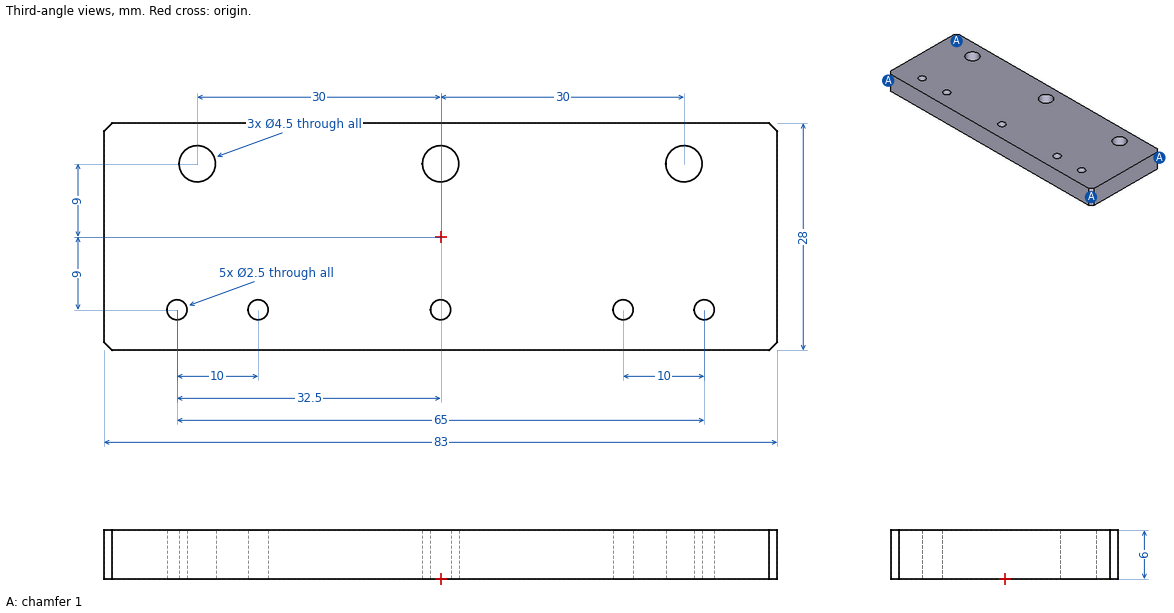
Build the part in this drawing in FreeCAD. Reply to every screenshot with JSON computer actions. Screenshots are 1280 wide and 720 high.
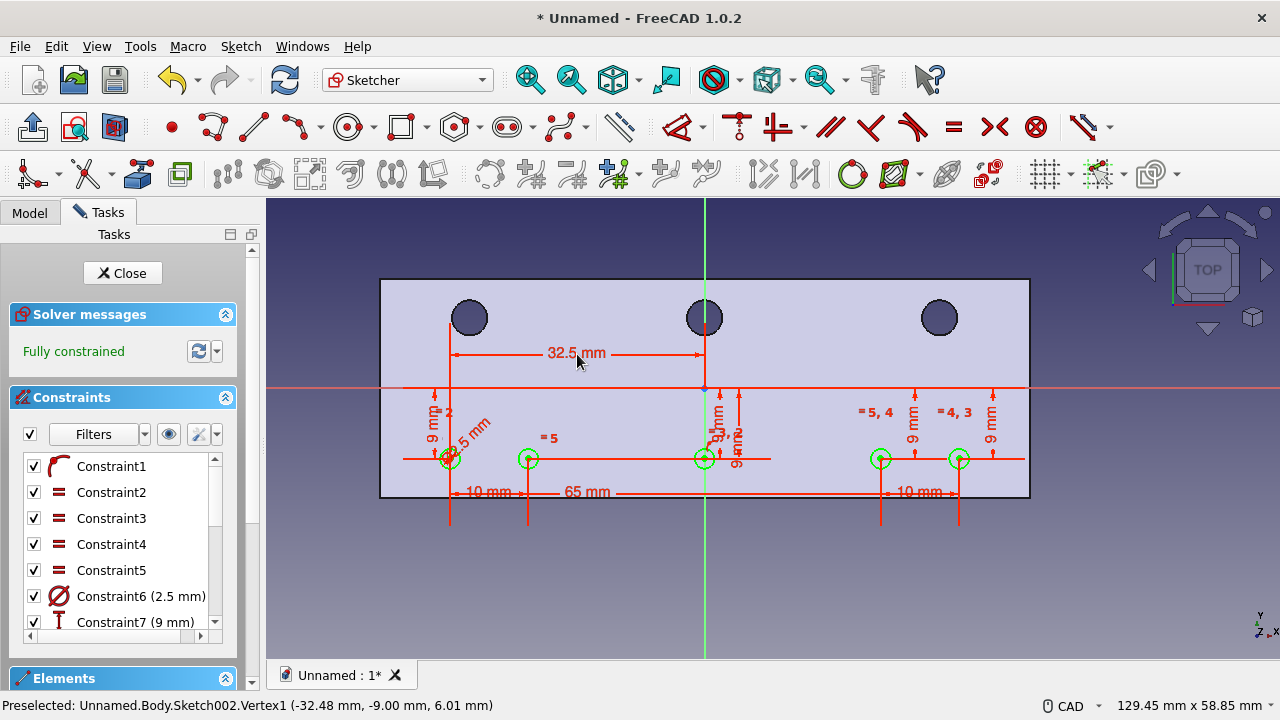
{"action": "left_click", "coordinate": [123, 273]}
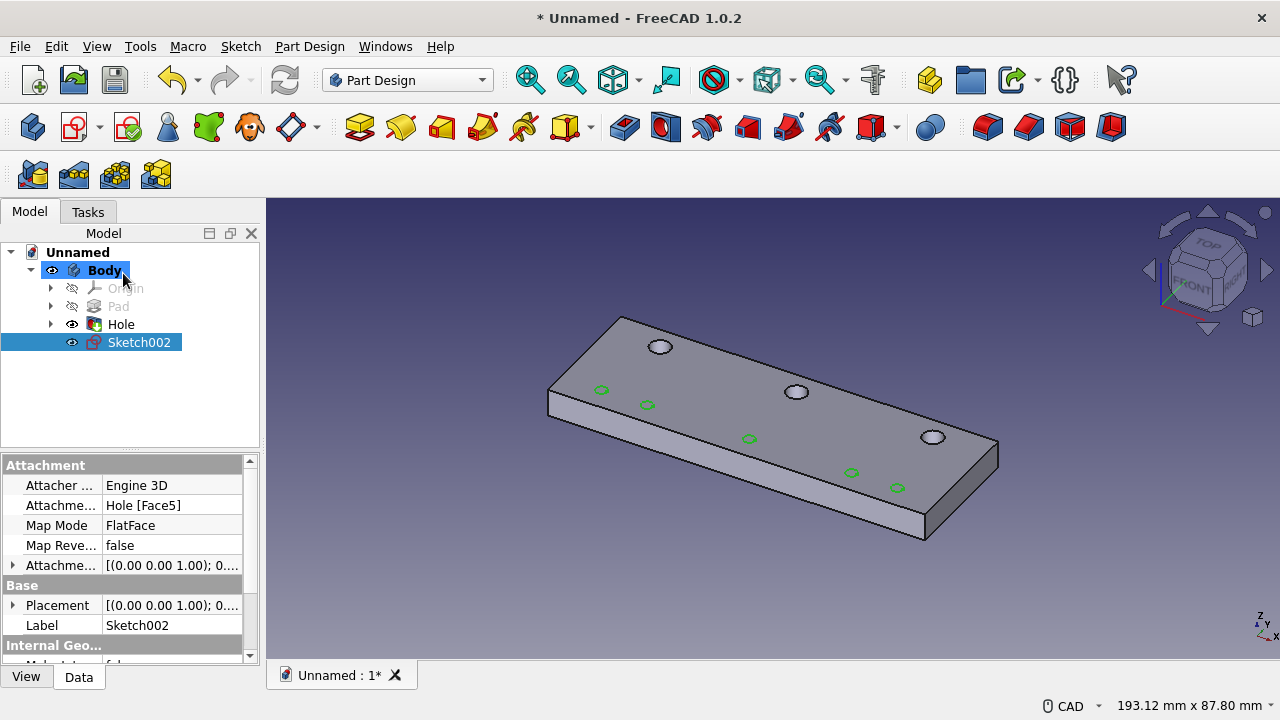
{"action": "left_click", "coordinate": [666, 128]}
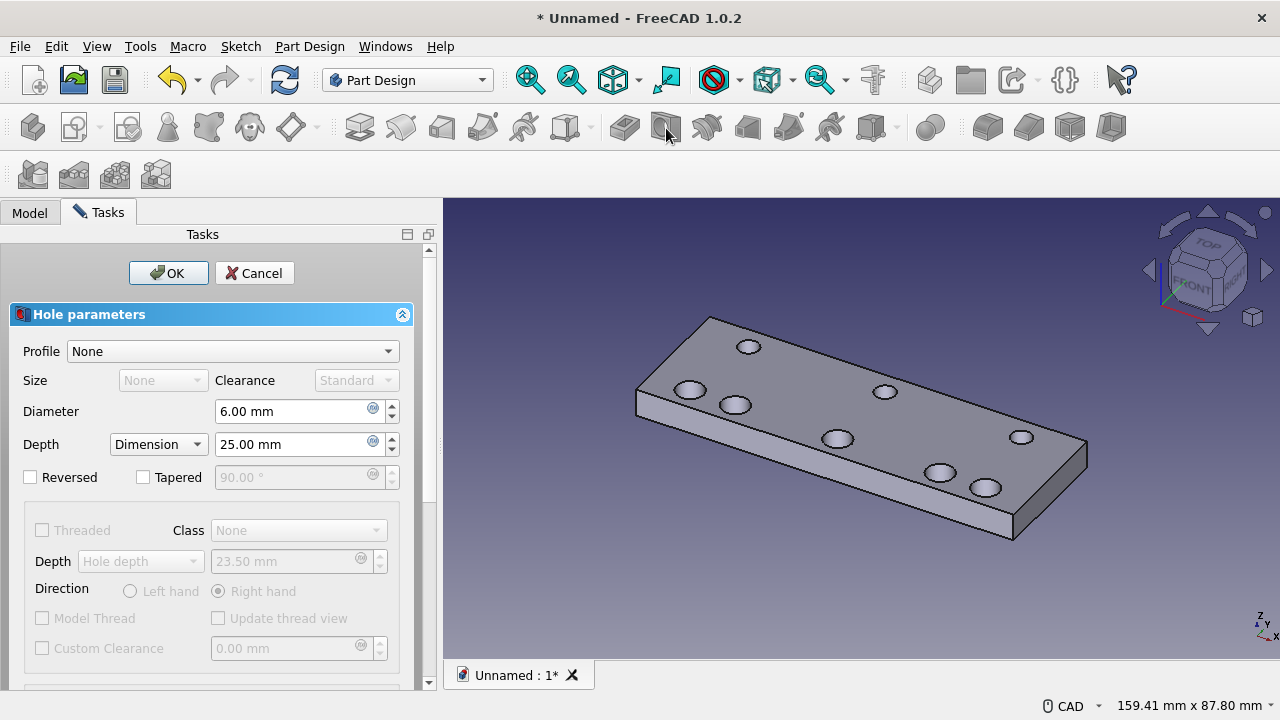
{"action": "triple_click", "coordinate": [300, 412]}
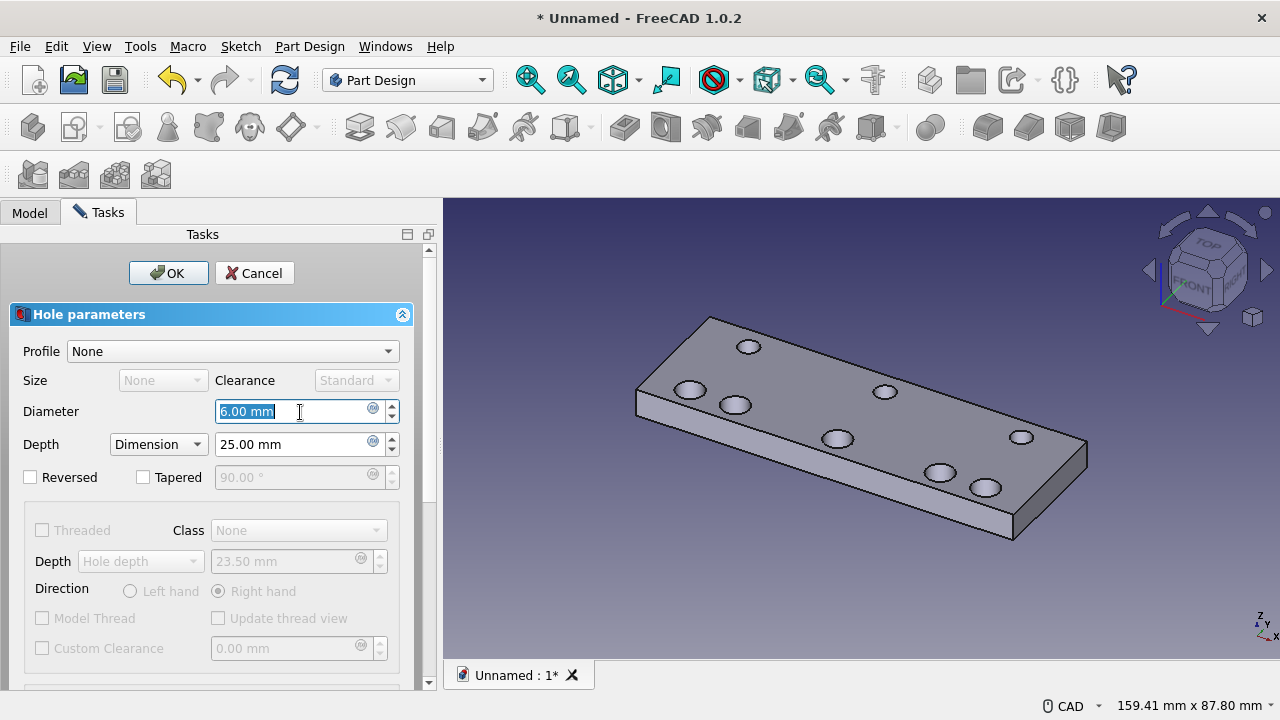
{"action": "type", "text": "2.5"}
{"action": "key", "text": "Tab"}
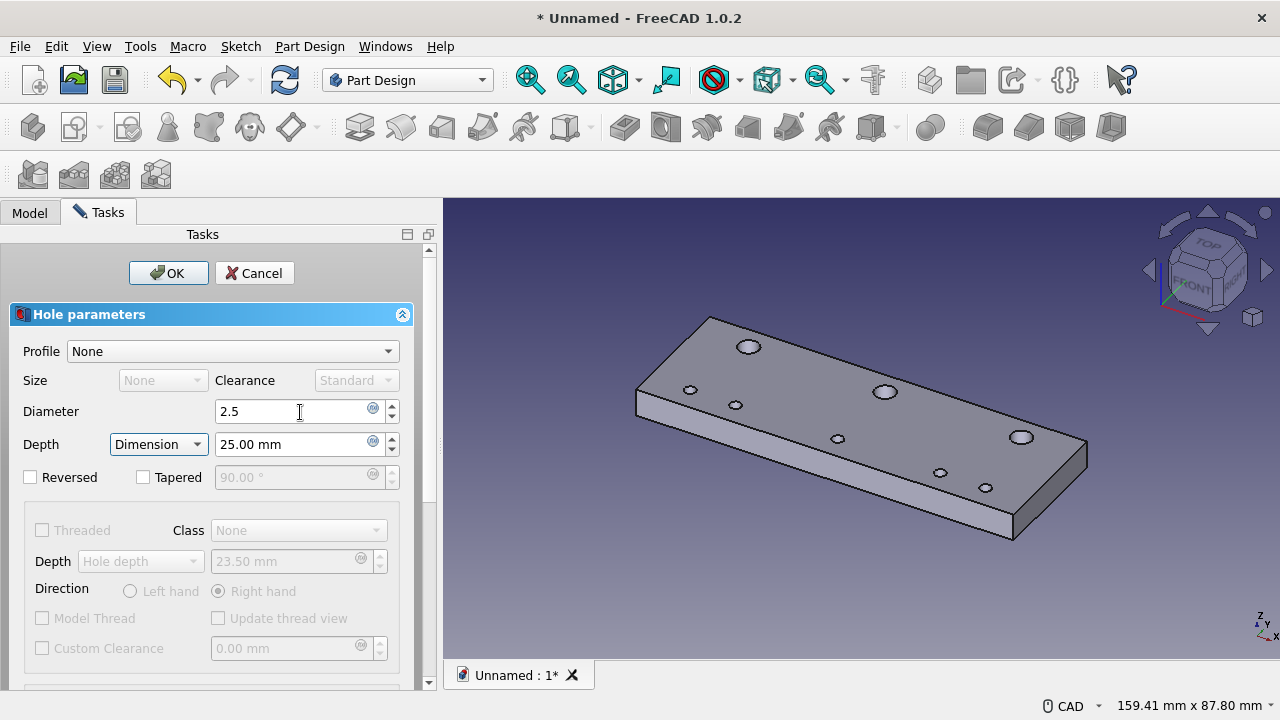
{"action": "left_click", "coordinate": [160, 444]}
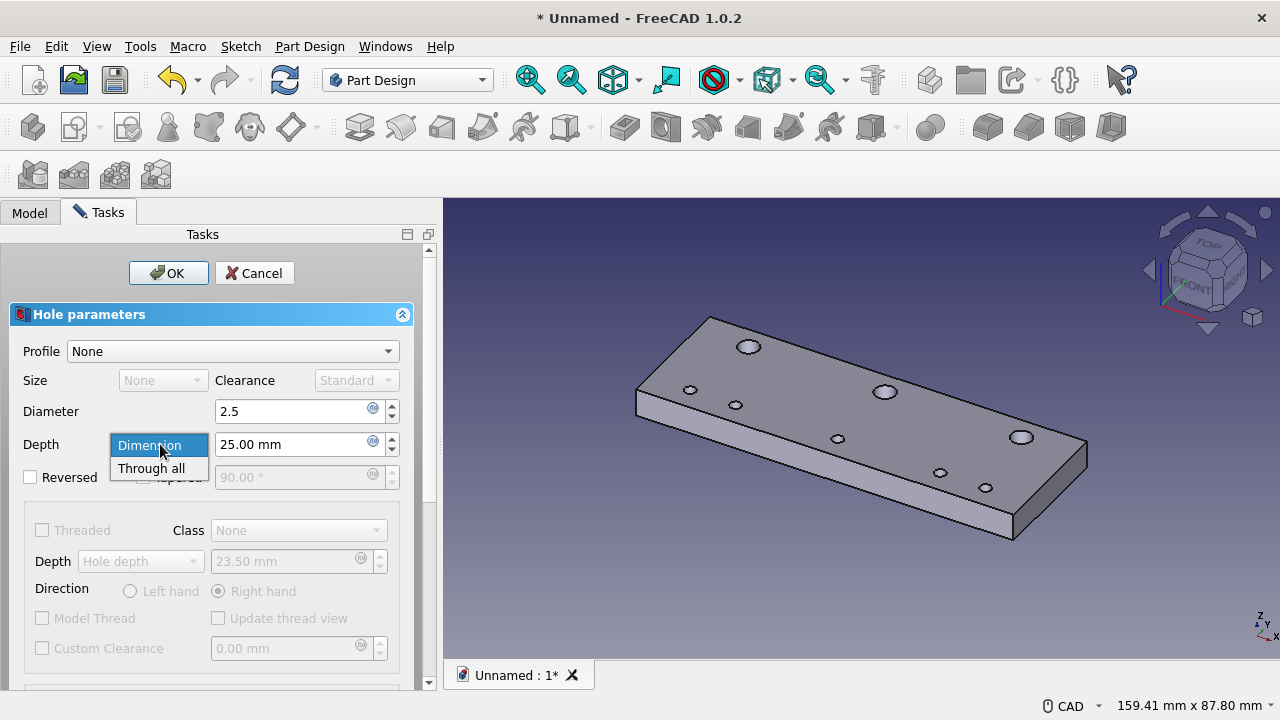
{"action": "left_click", "coordinate": [158, 468]}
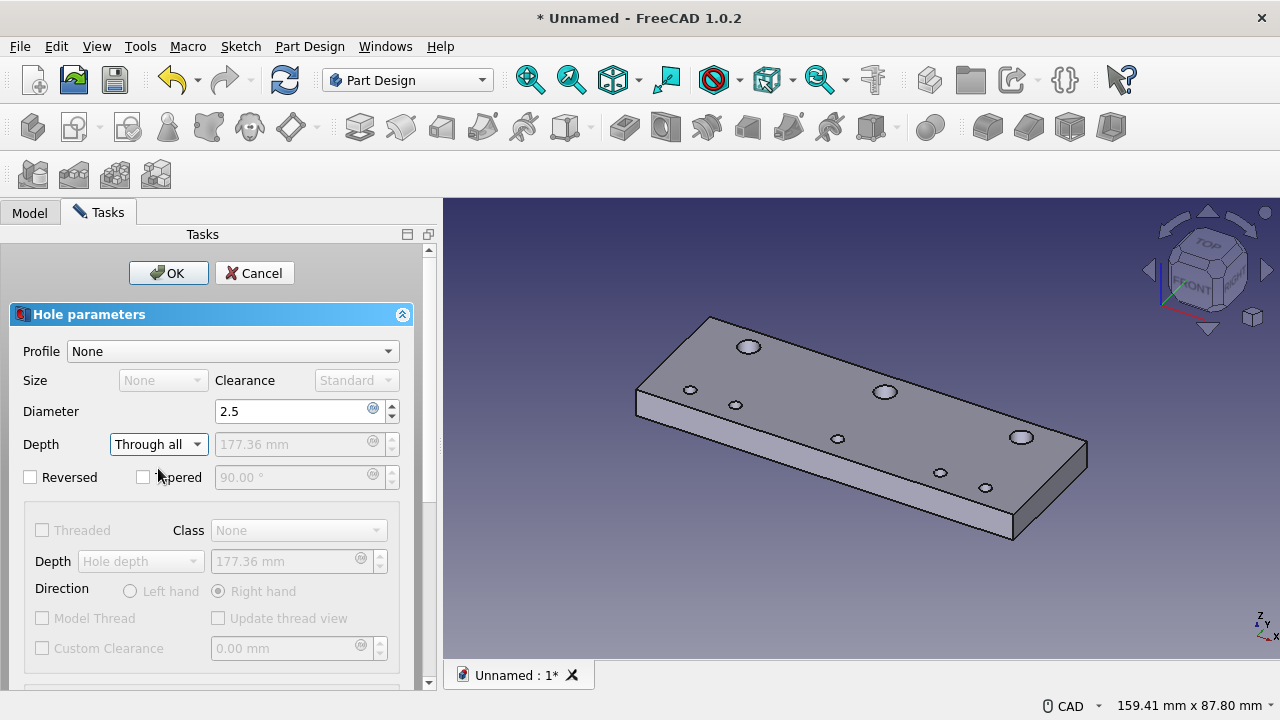
{"action": "left_click", "coordinate": [169, 273]}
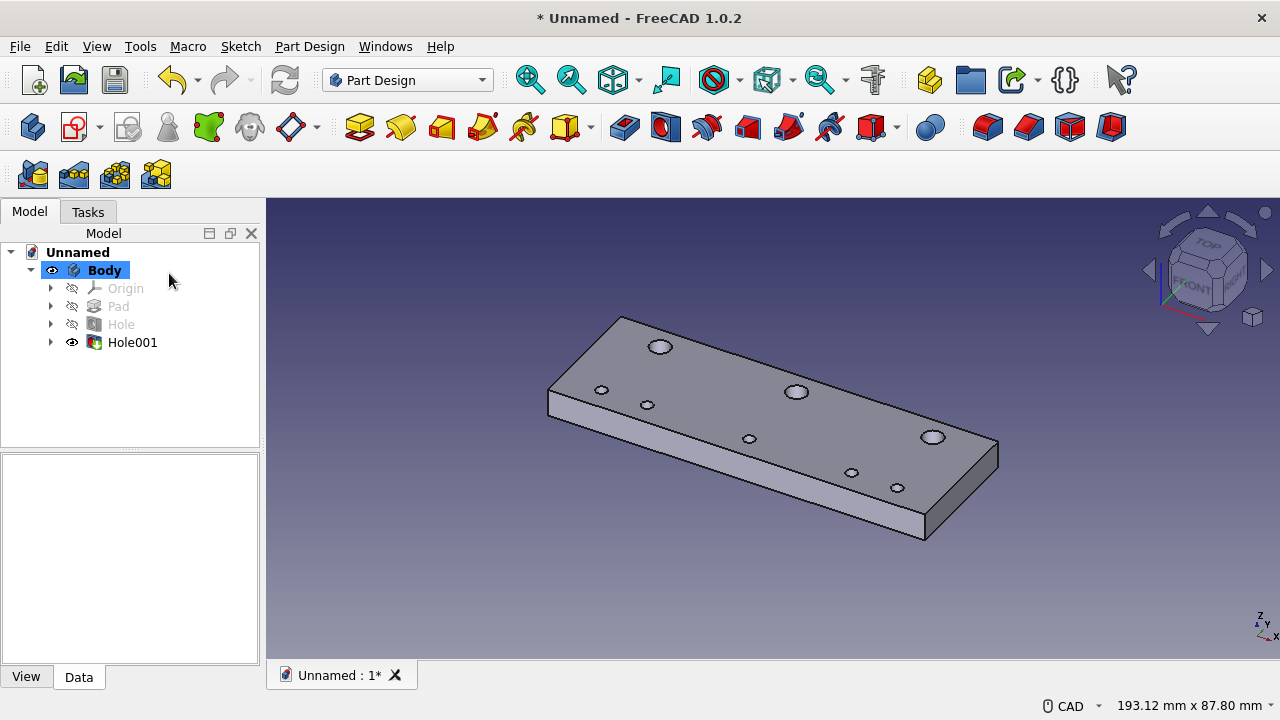
{"action": "left_click", "coordinate": [925, 527]}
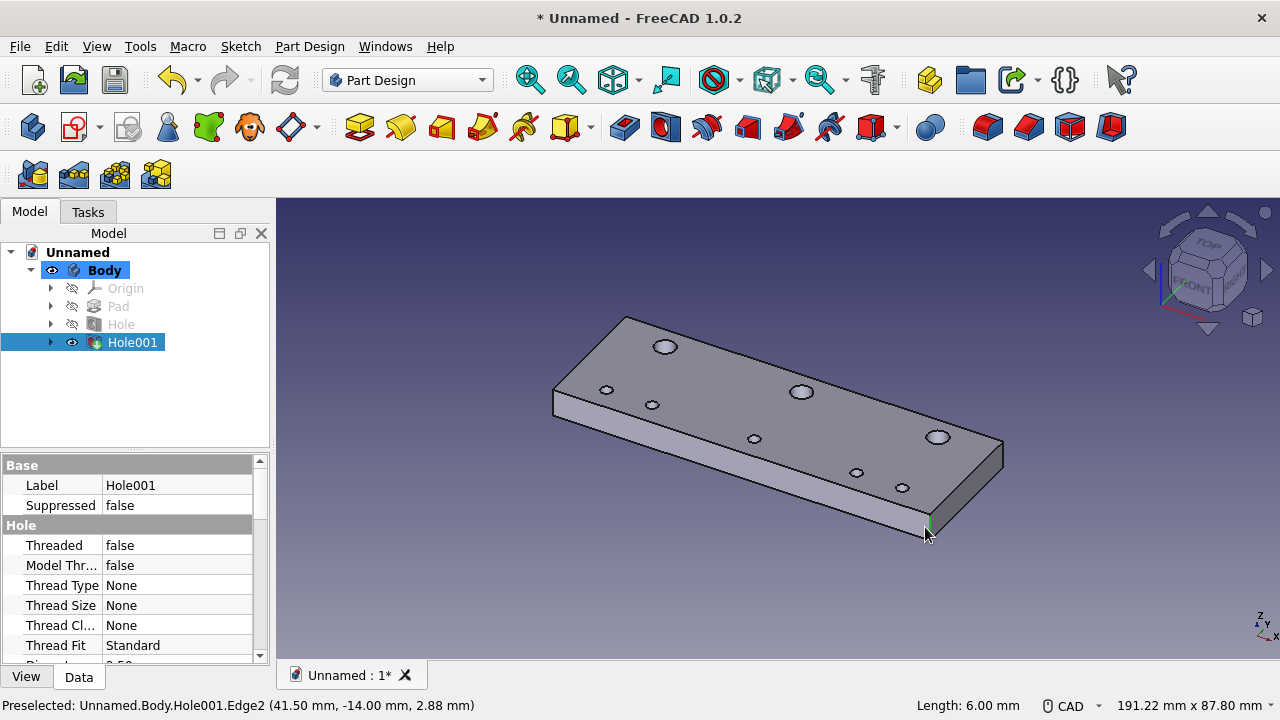
{"action": "key", "text": "0"}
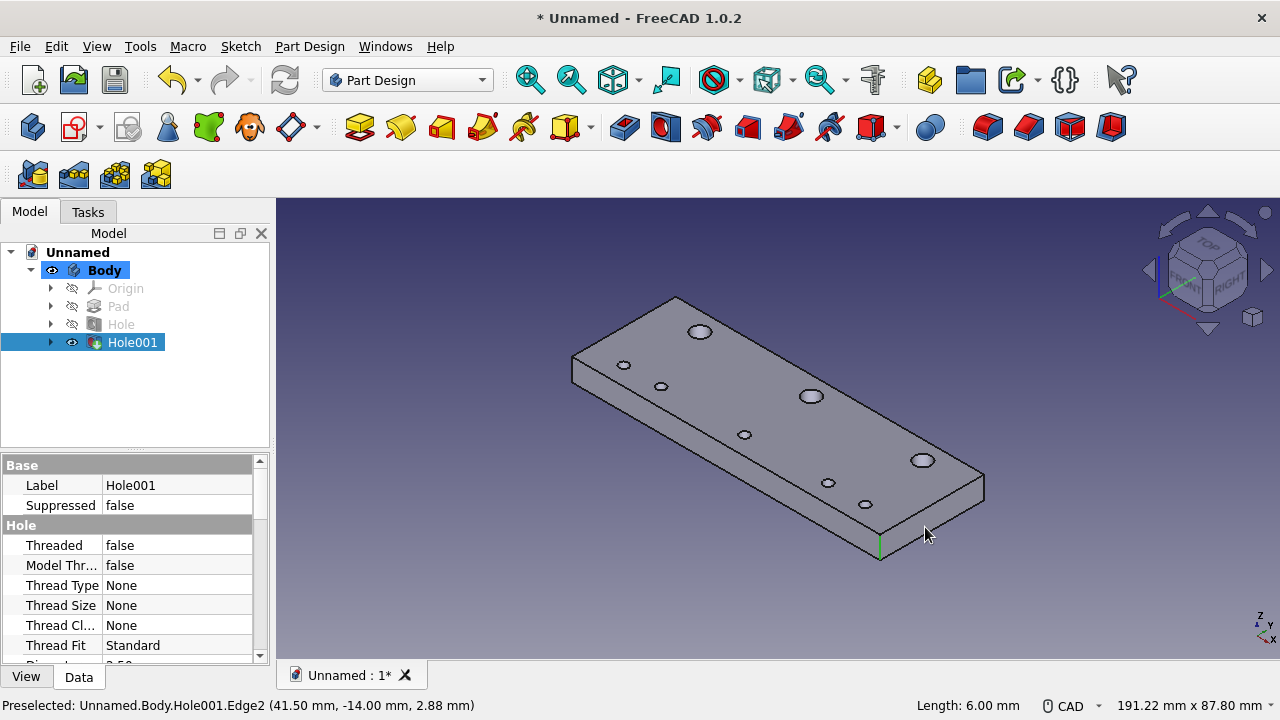
{"action": "key", "text": "2"}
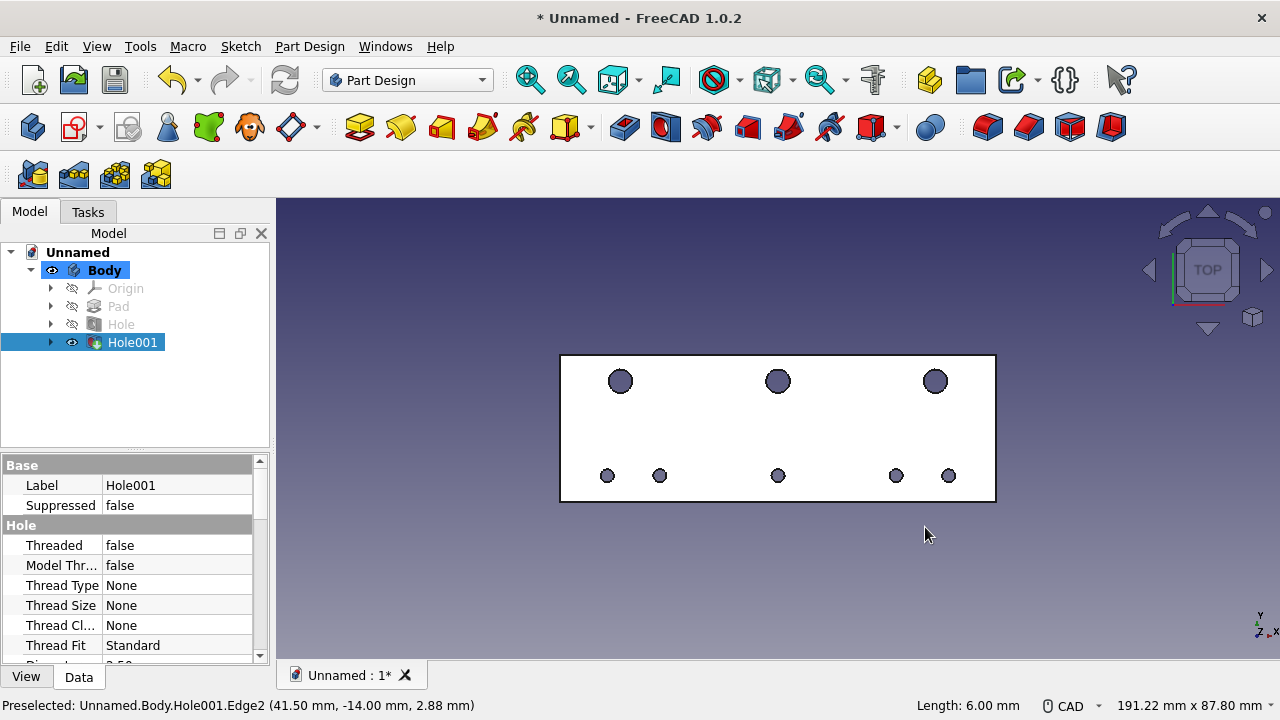
{"action": "key", "text": "v f"}